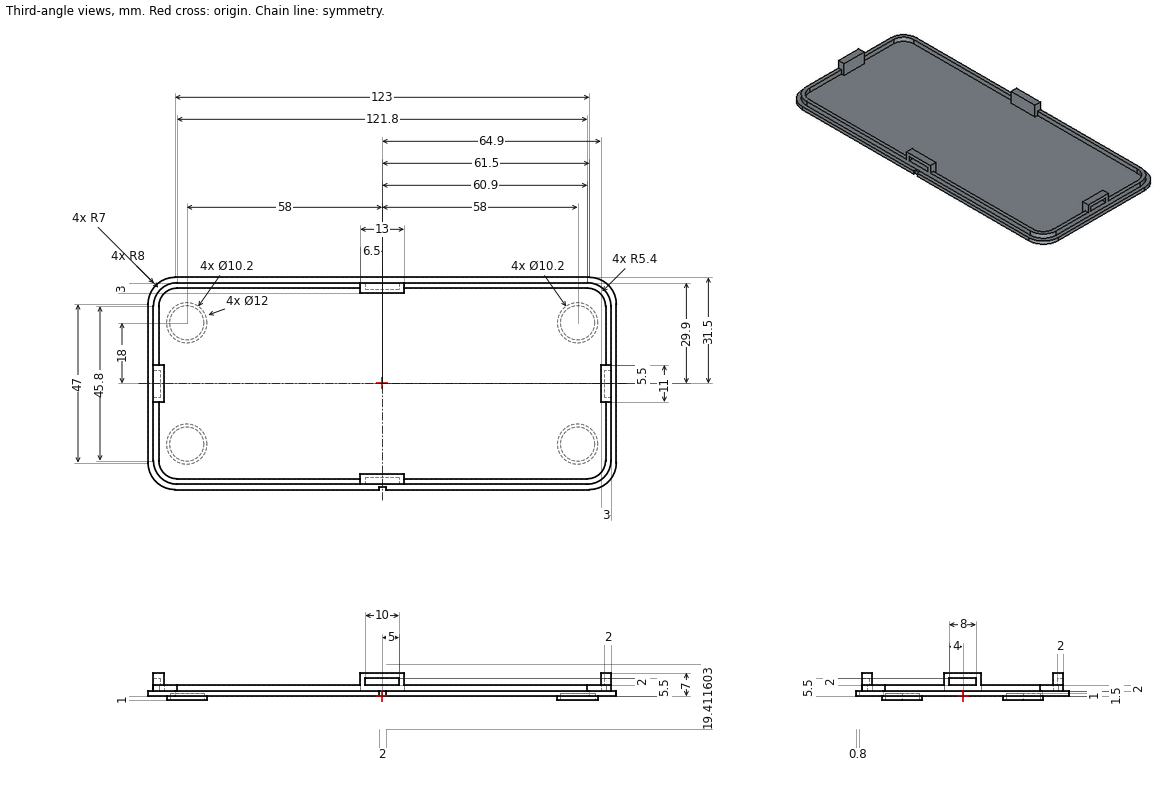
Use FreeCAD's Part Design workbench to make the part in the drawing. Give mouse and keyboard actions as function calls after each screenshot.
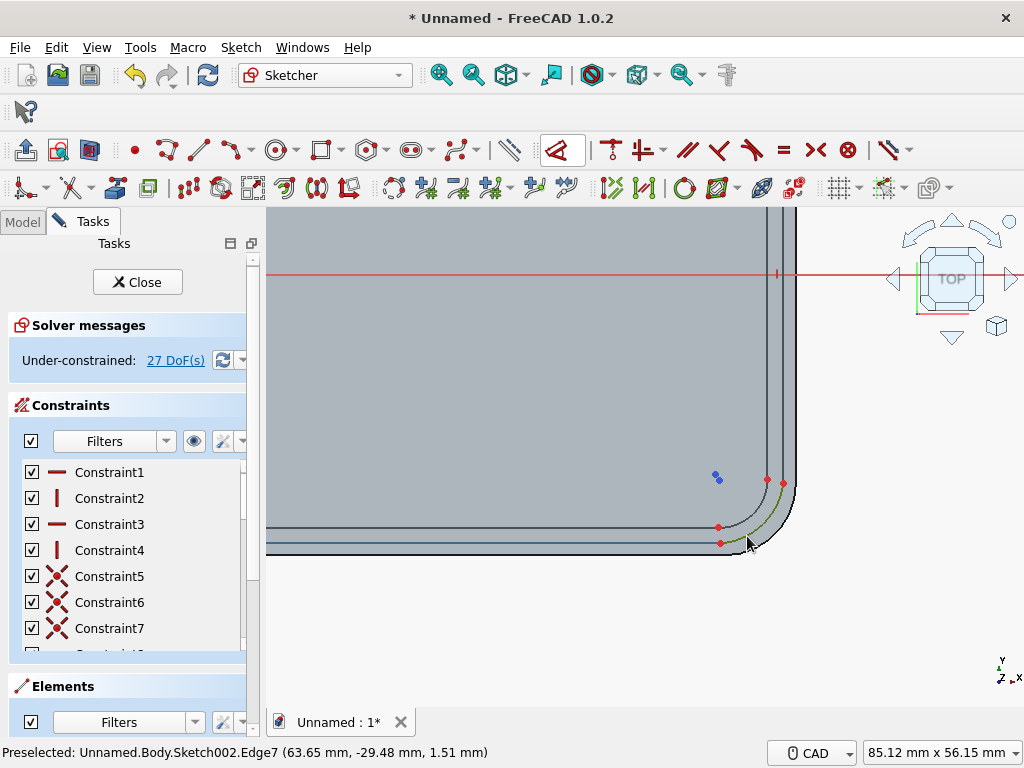
key(t)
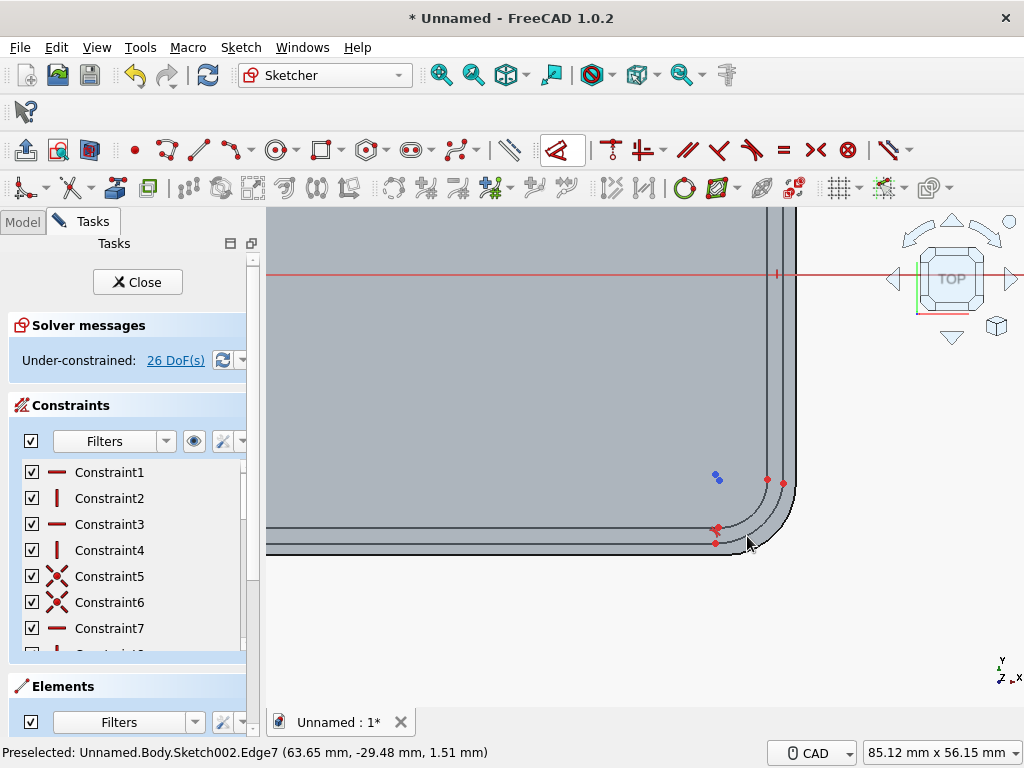
click(783, 361)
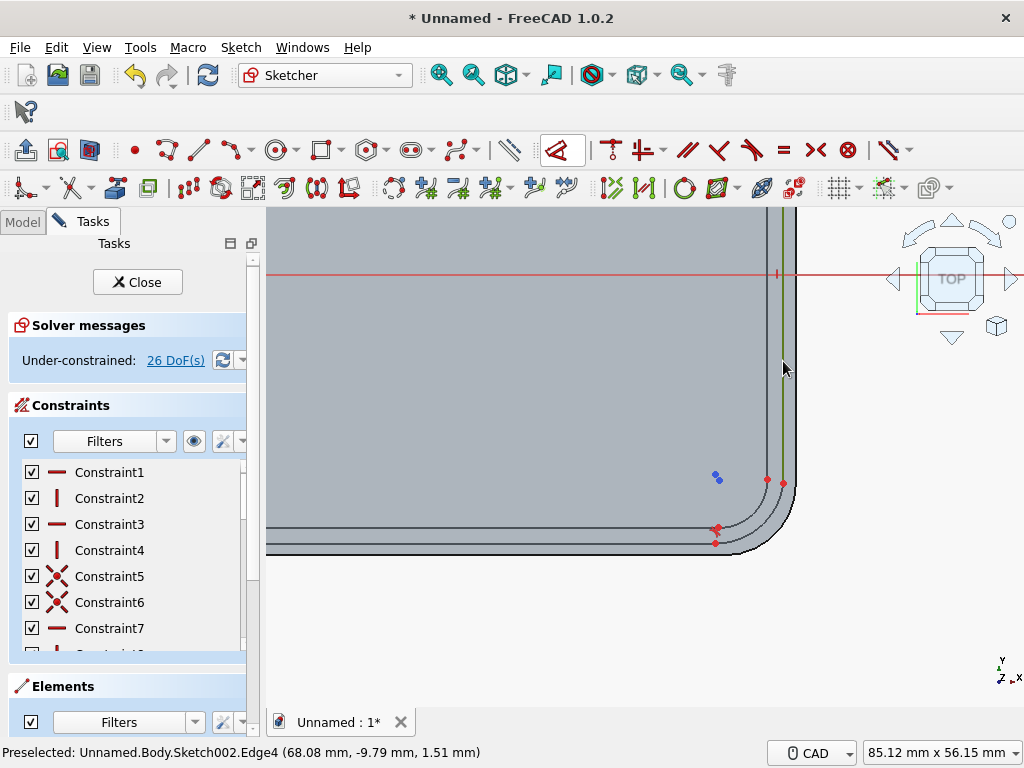
click(744, 537)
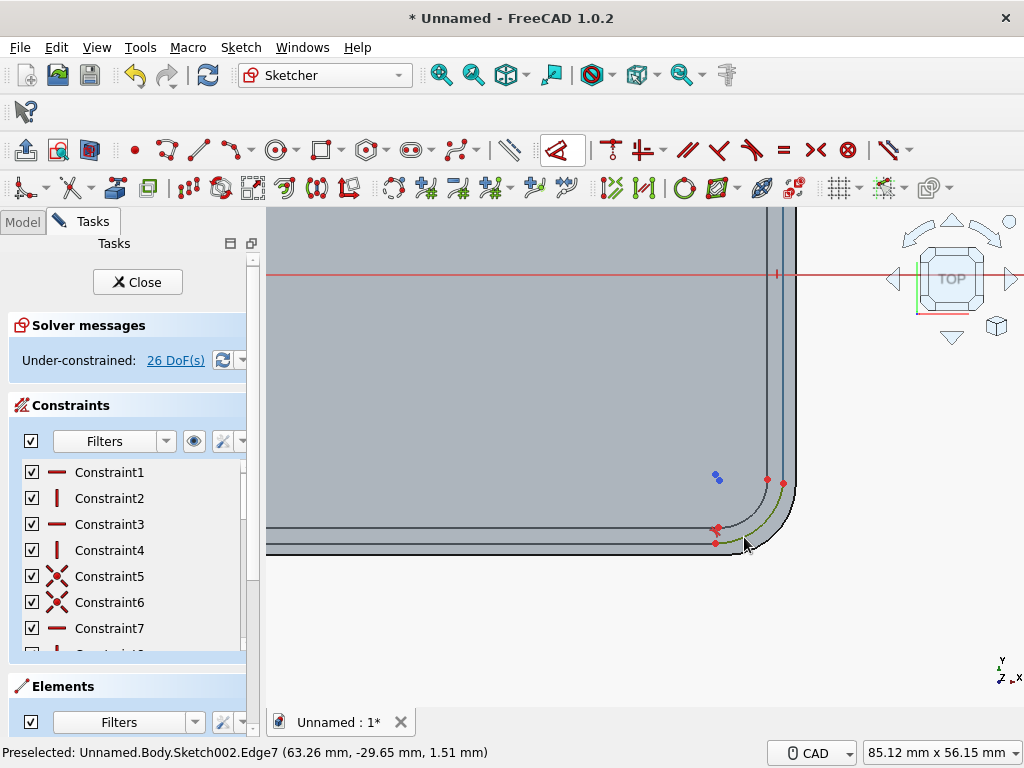
key(t)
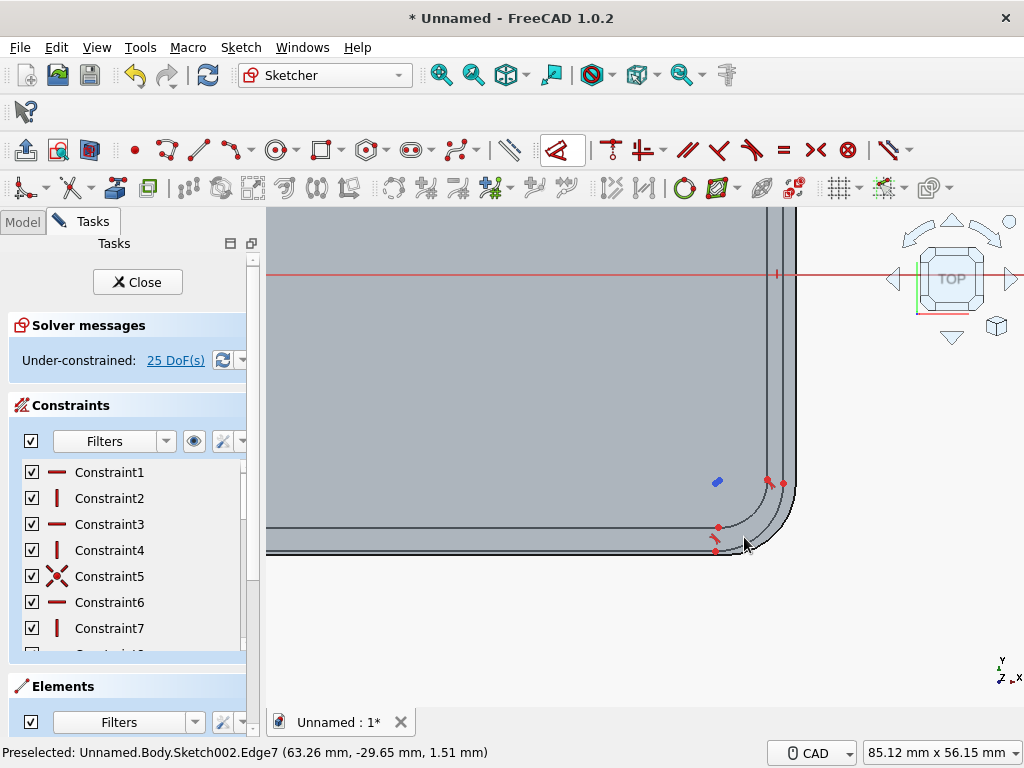
click(783, 361)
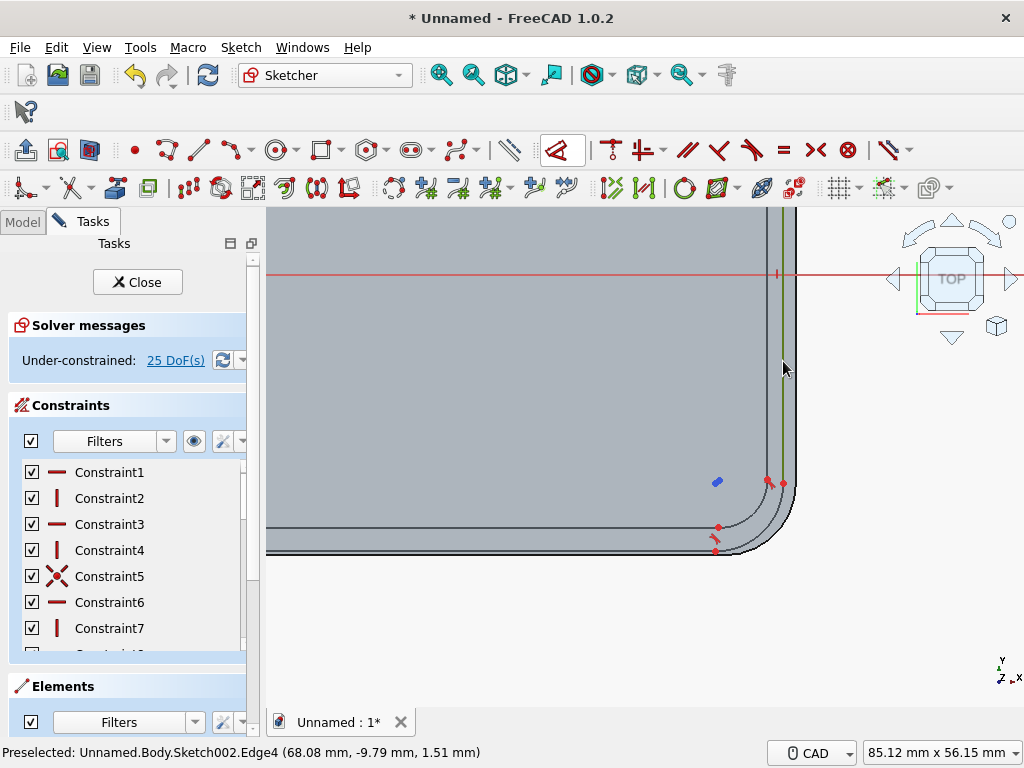
scroll(749, 536, down, 6)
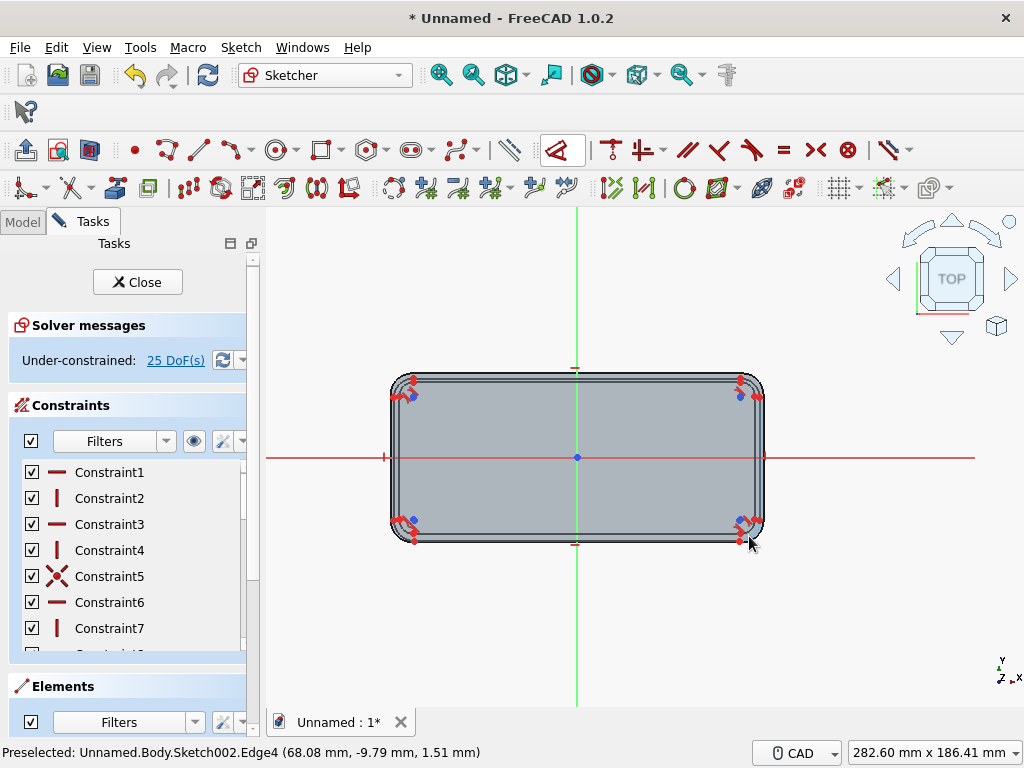
scroll(758, 389, up, 6)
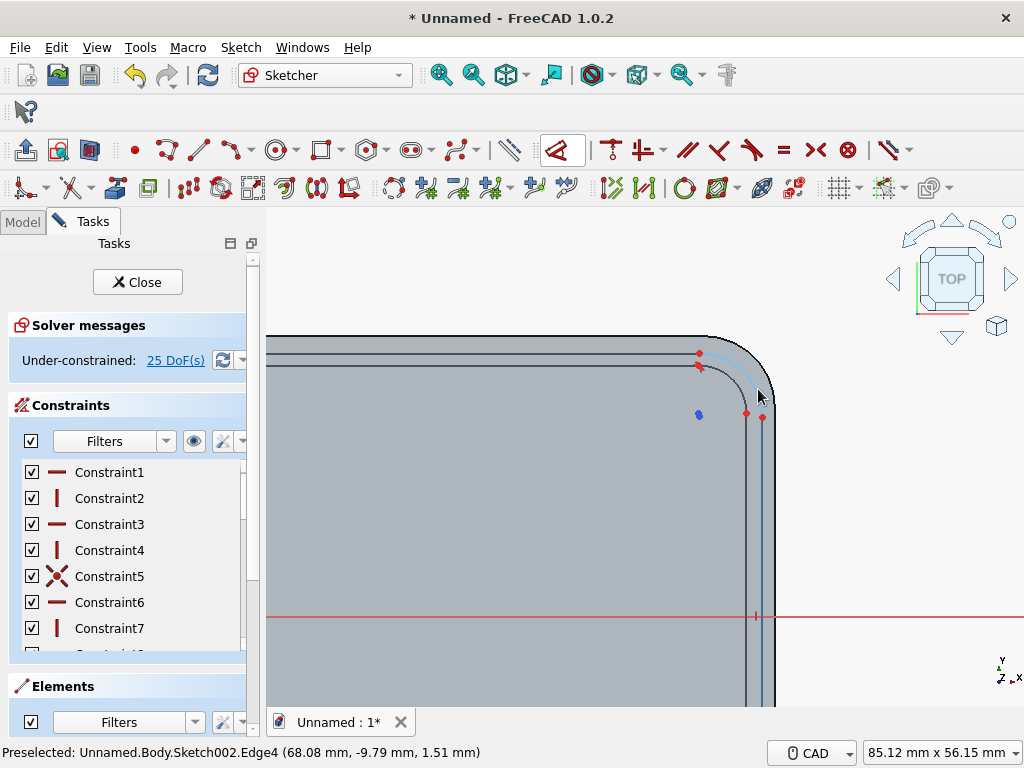
click(755, 388)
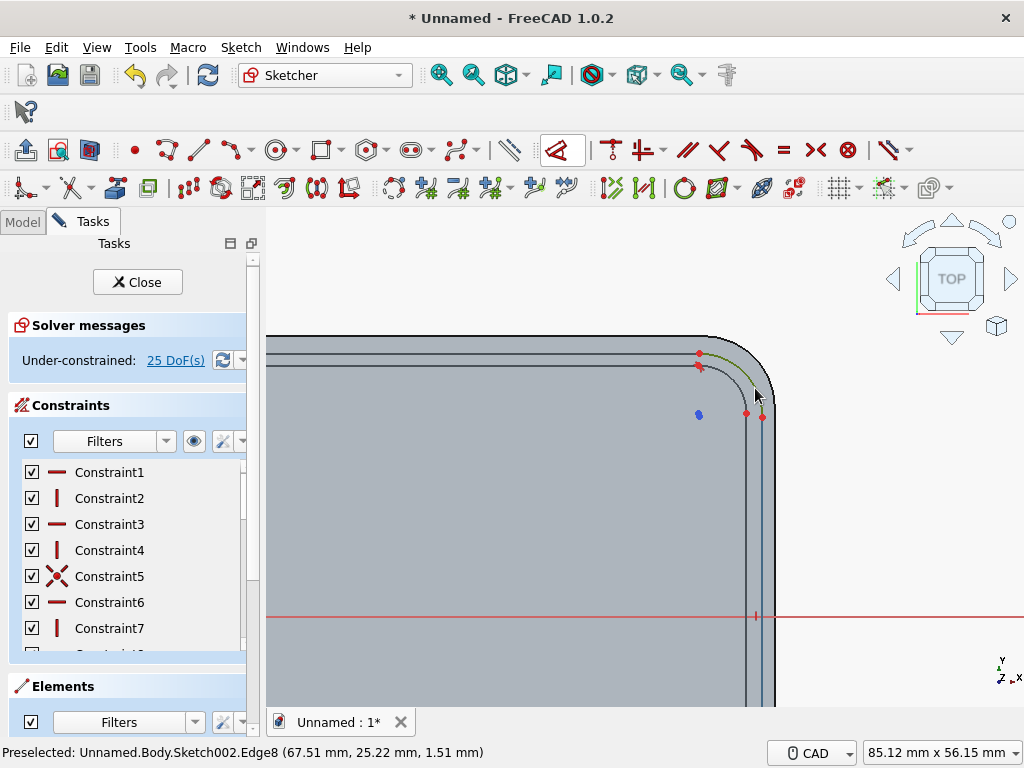
click(752, 150)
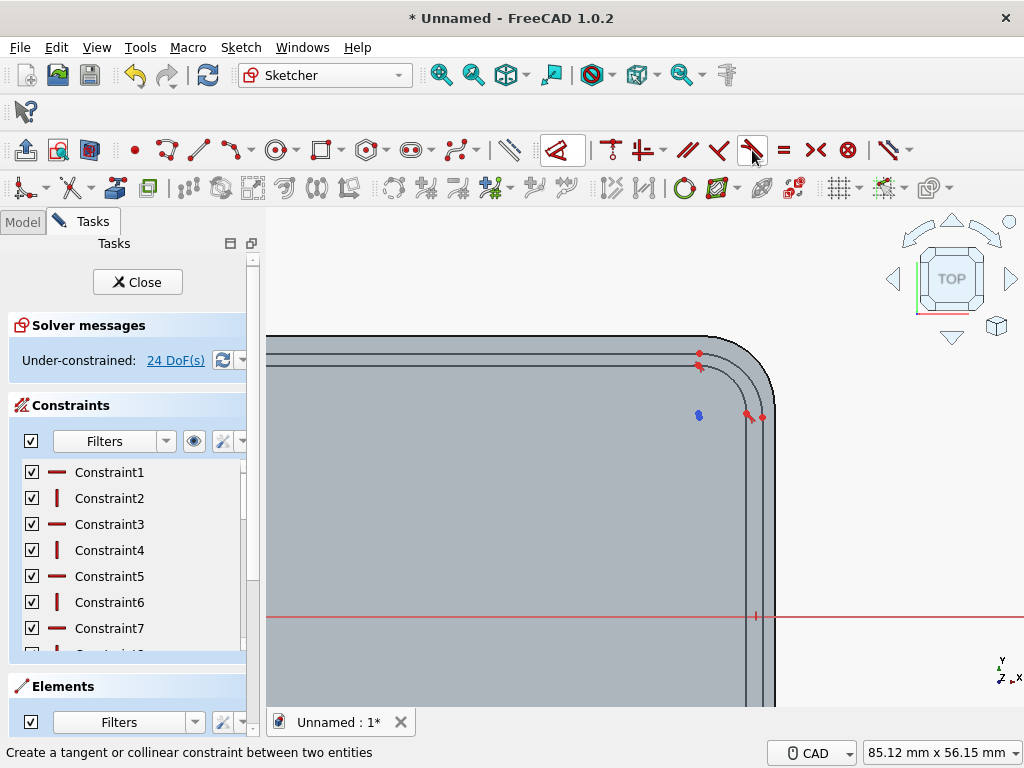
click(373, 366)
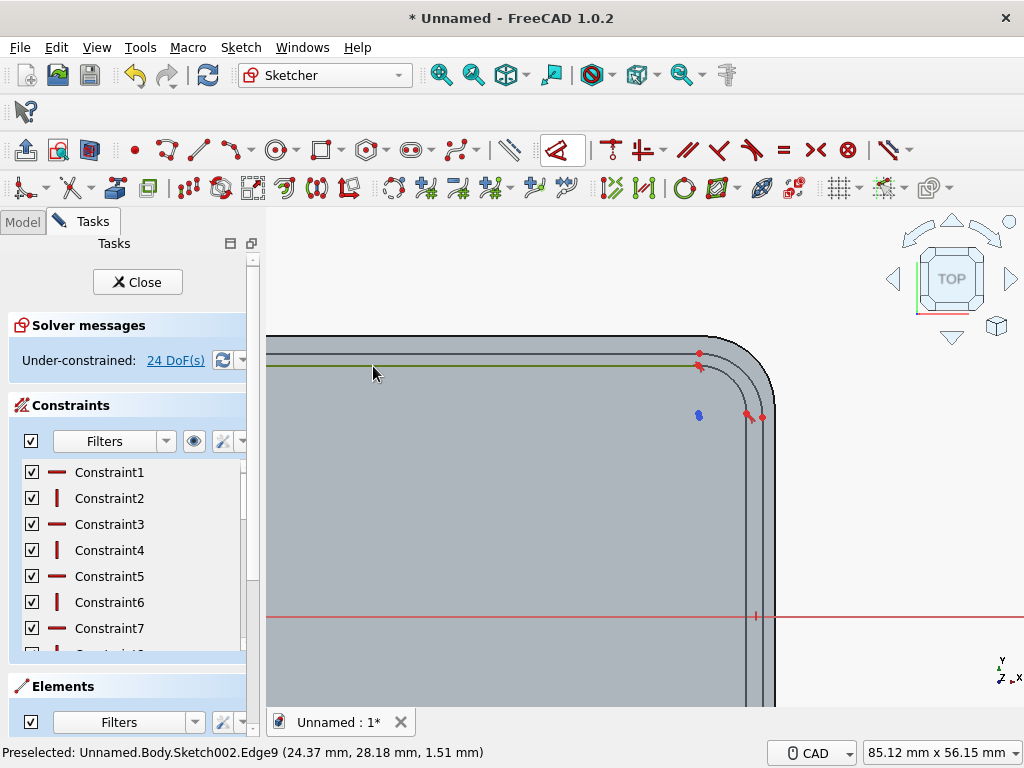
click(741, 391)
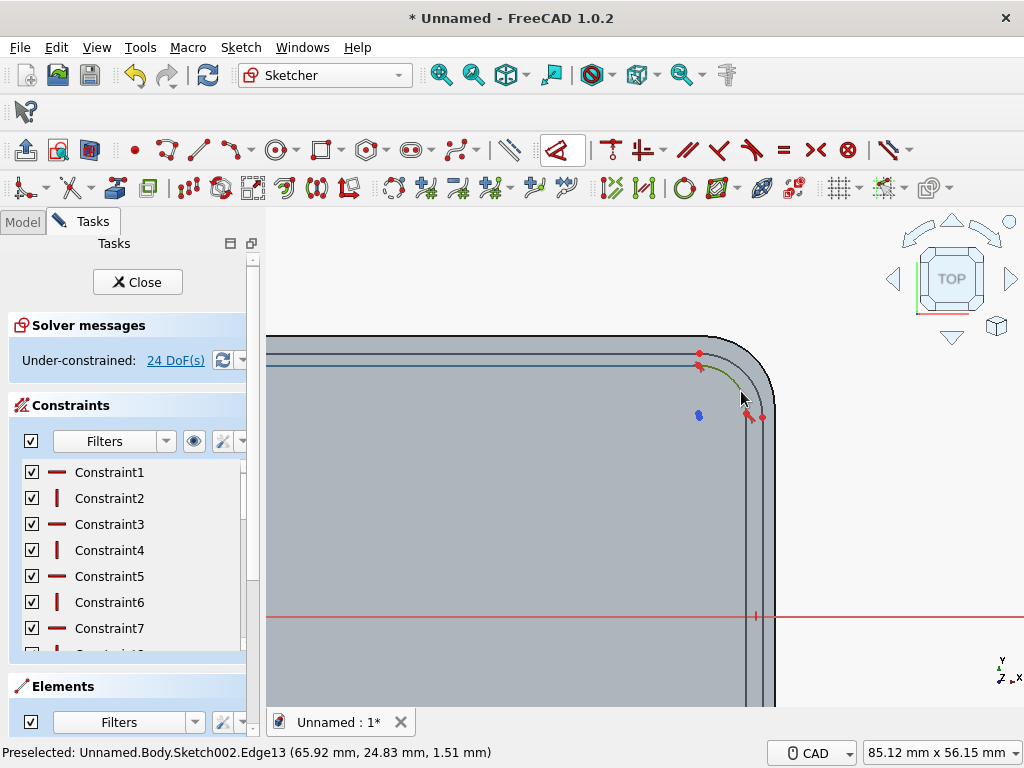
key(t)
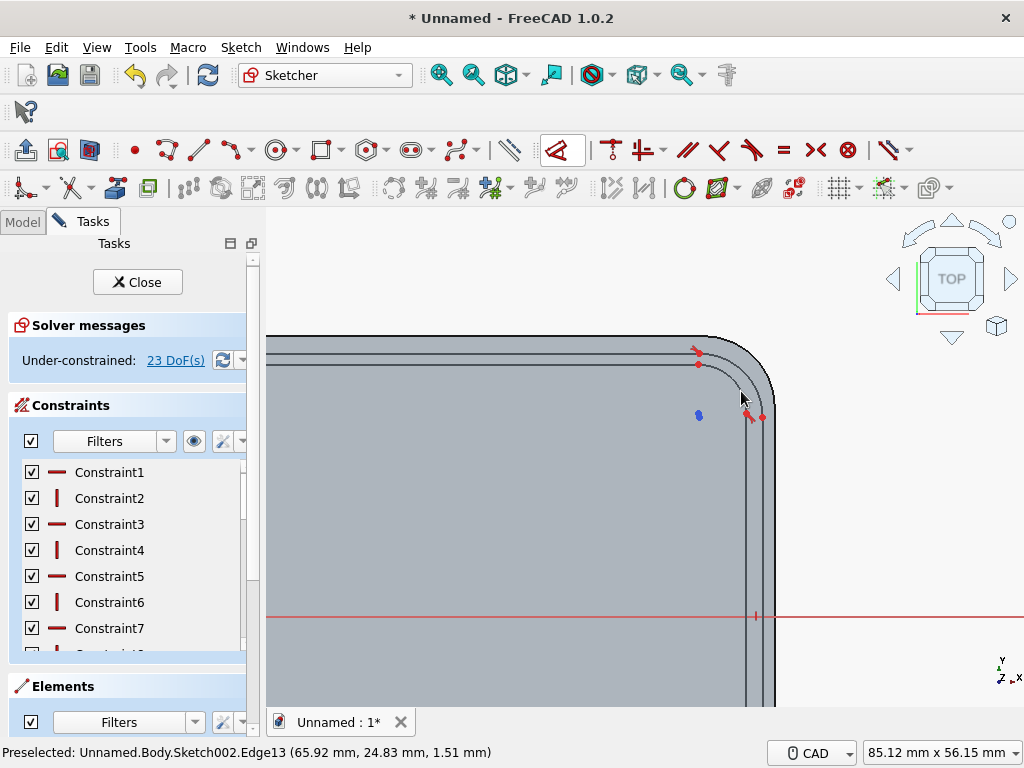
scroll(373, 365, up, 2)